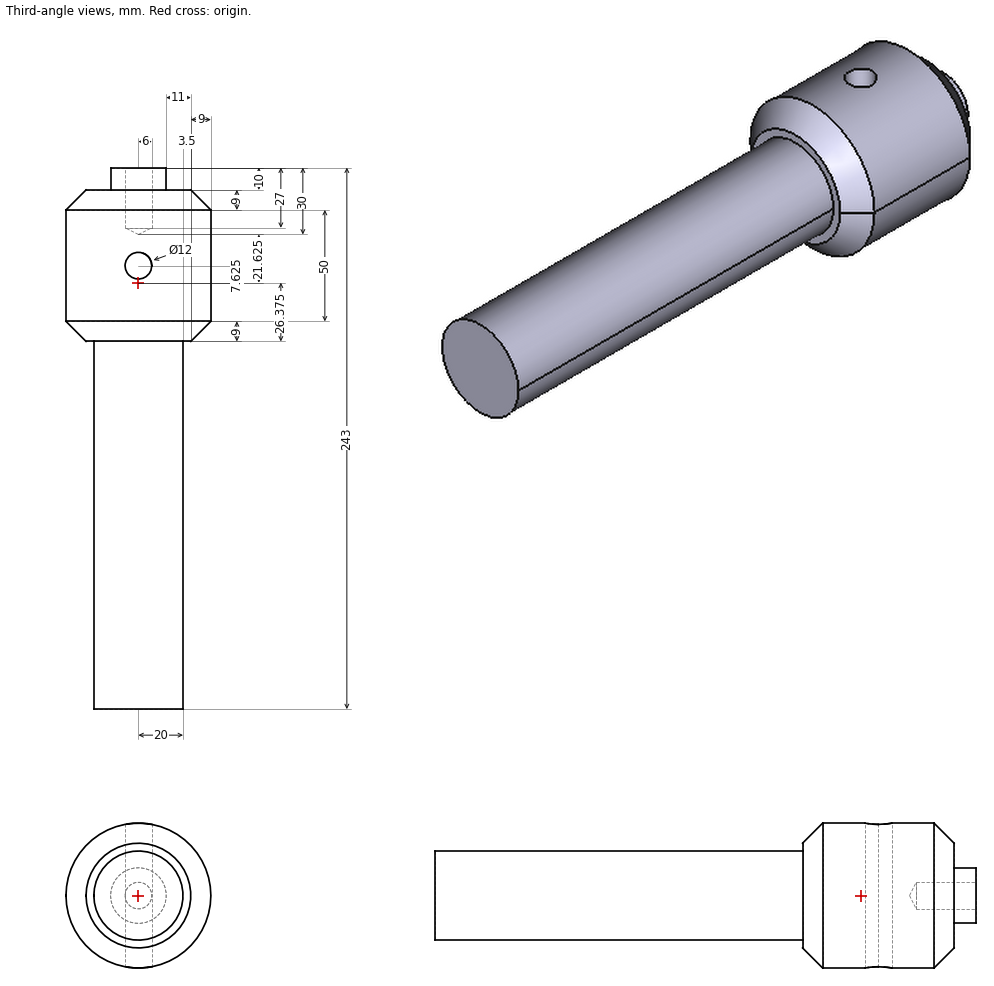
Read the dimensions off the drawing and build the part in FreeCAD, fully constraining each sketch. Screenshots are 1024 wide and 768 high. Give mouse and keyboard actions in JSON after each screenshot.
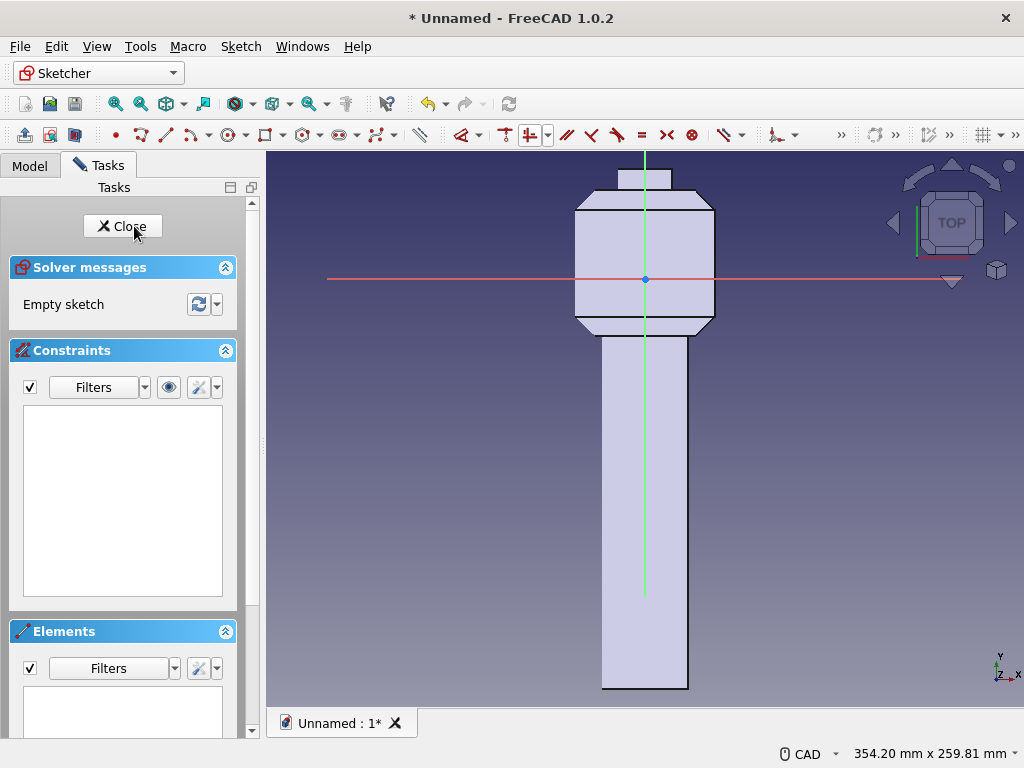
{"action": "scroll", "coordinate": [576, 429], "scroll_direction": "down", "scroll_amount": 5}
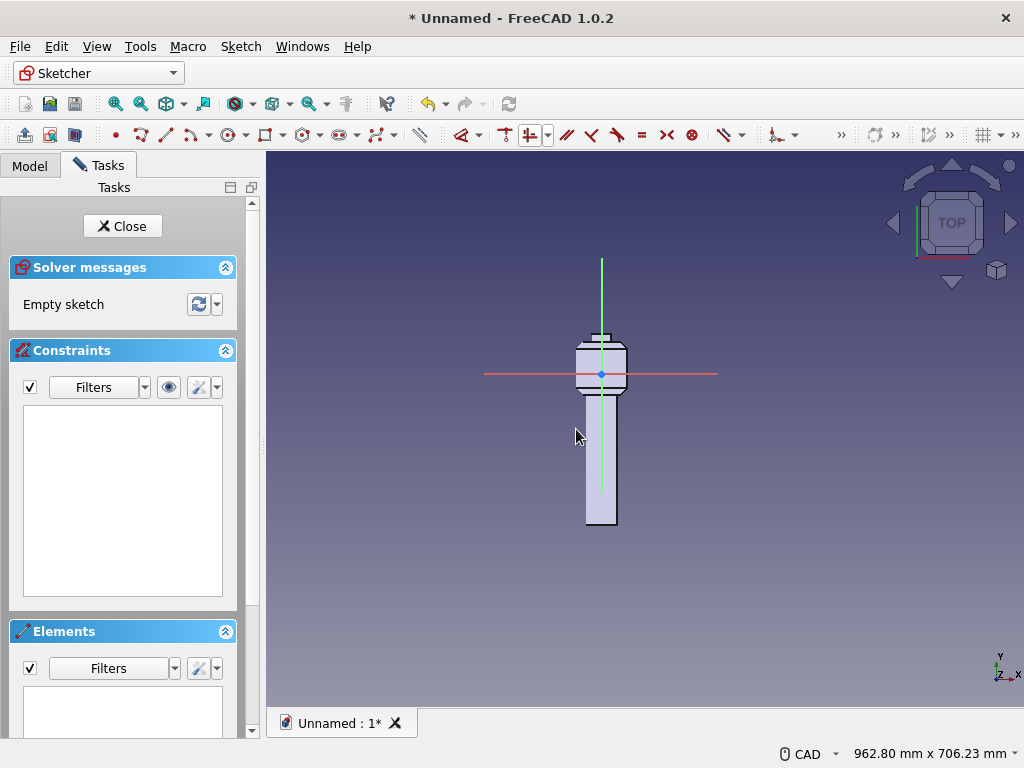
{"action": "scroll", "coordinate": [607, 345], "scroll_direction": "up", "scroll_amount": 11}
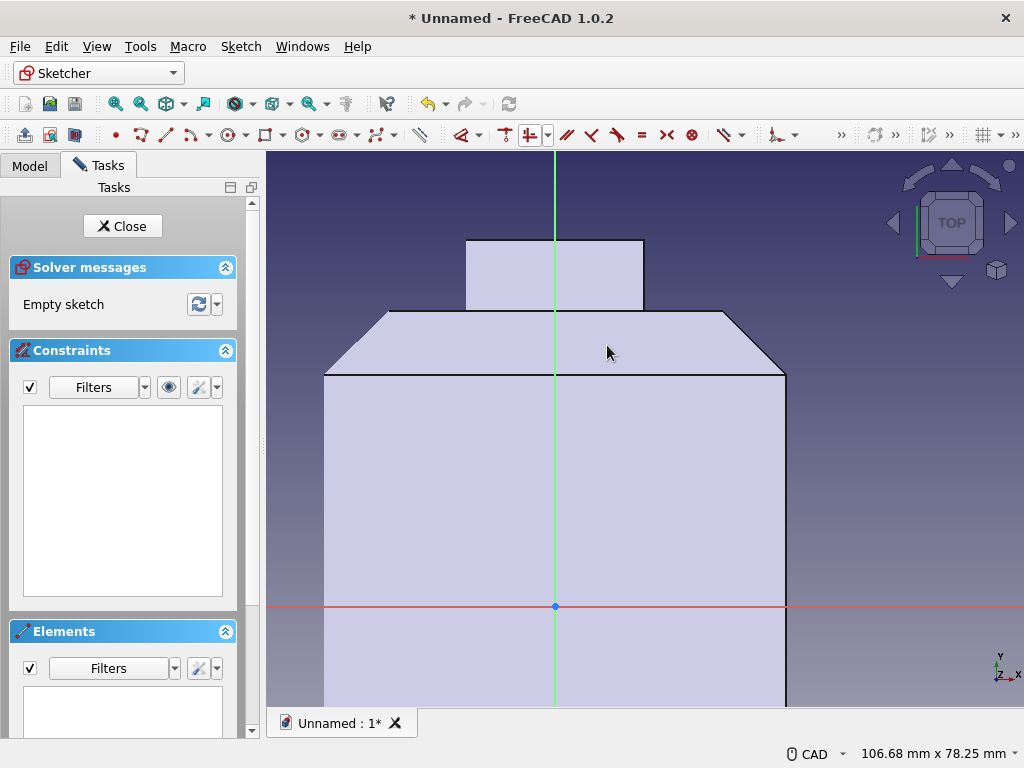
{"action": "left_click", "coordinate": [141, 136]}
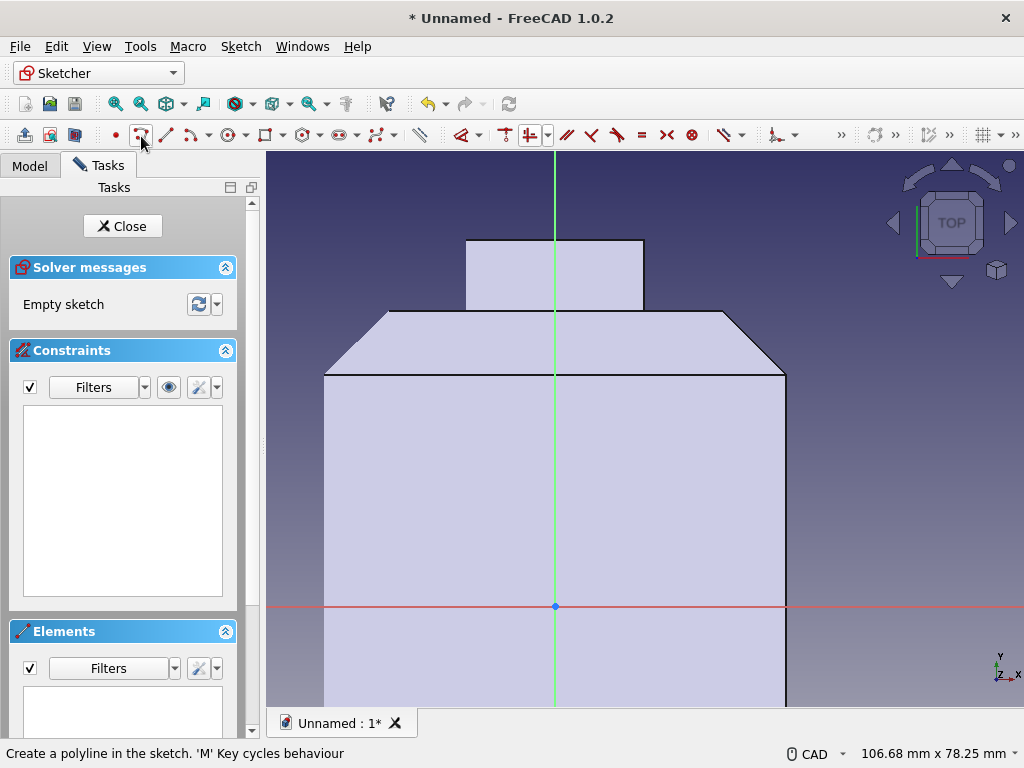
{"action": "left_click", "coordinate": [555, 453]}
{"action": "left_click", "coordinate": [598, 432]}
{"action": "left_click", "coordinate": [598, 240]}
{"action": "left_click", "coordinate": [564, 240]}
{"action": "left_click", "coordinate": [555, 454]}
{"action": "key", "text": "Escape"}
{"action": "key", "text": "Escape"}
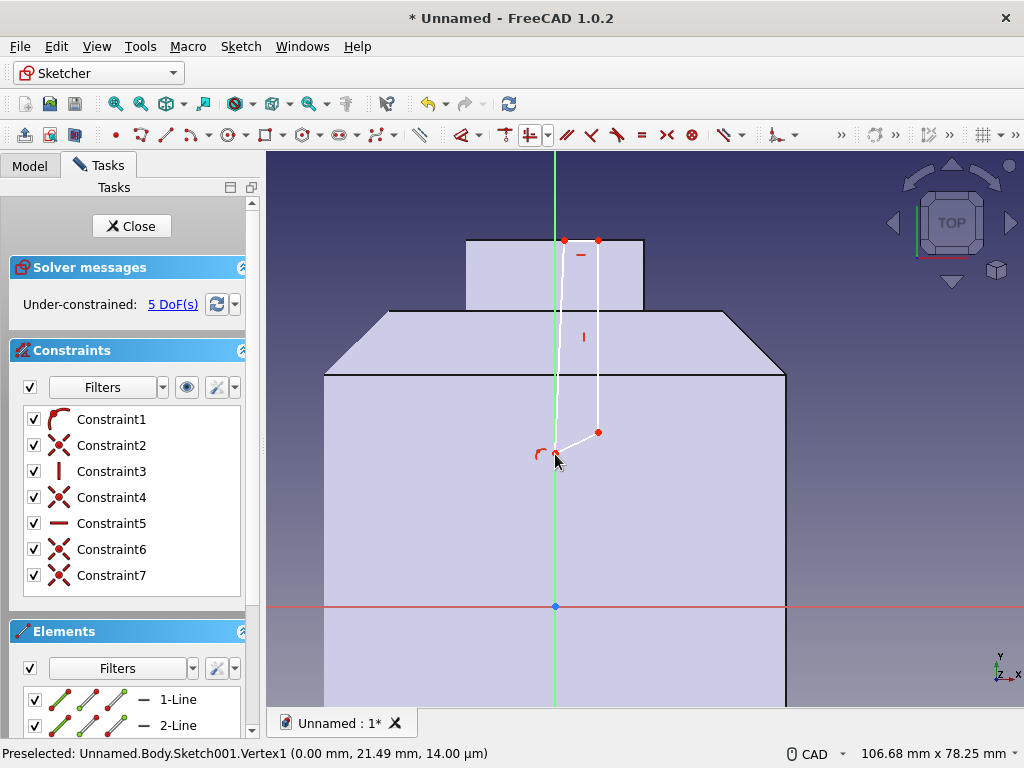
{"action": "left_click", "coordinate": [558, 390]}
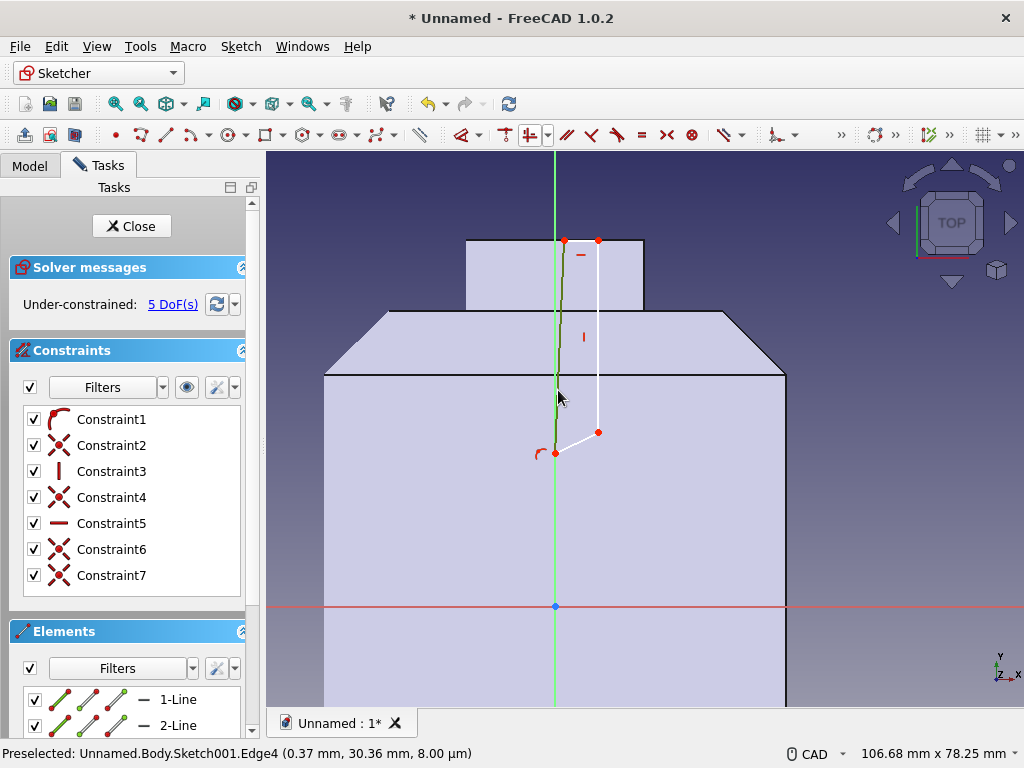
{"action": "left_click", "coordinate": [548, 136]}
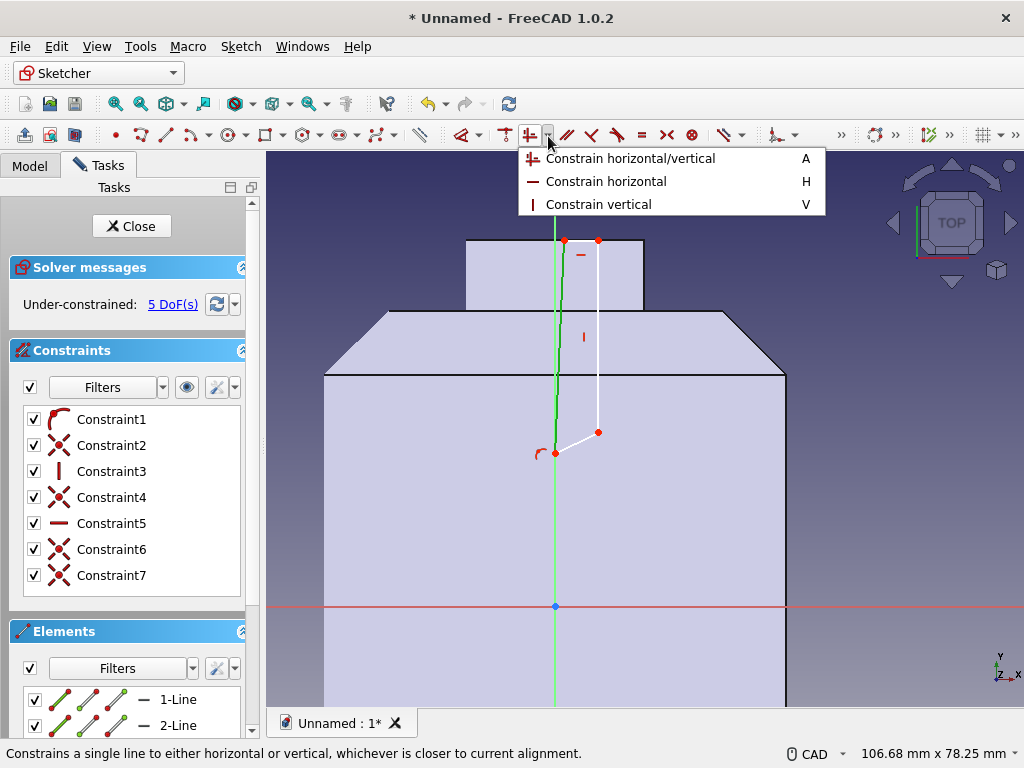
{"action": "left_click", "coordinate": [672, 204]}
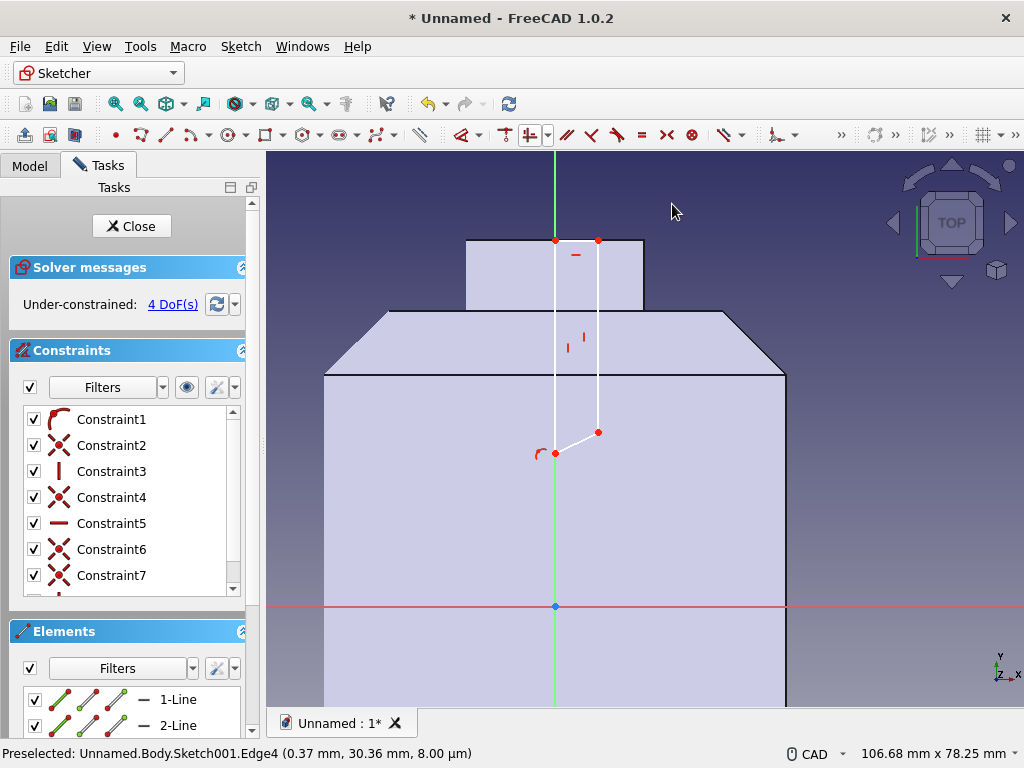
{"action": "left_click", "coordinate": [460, 136]}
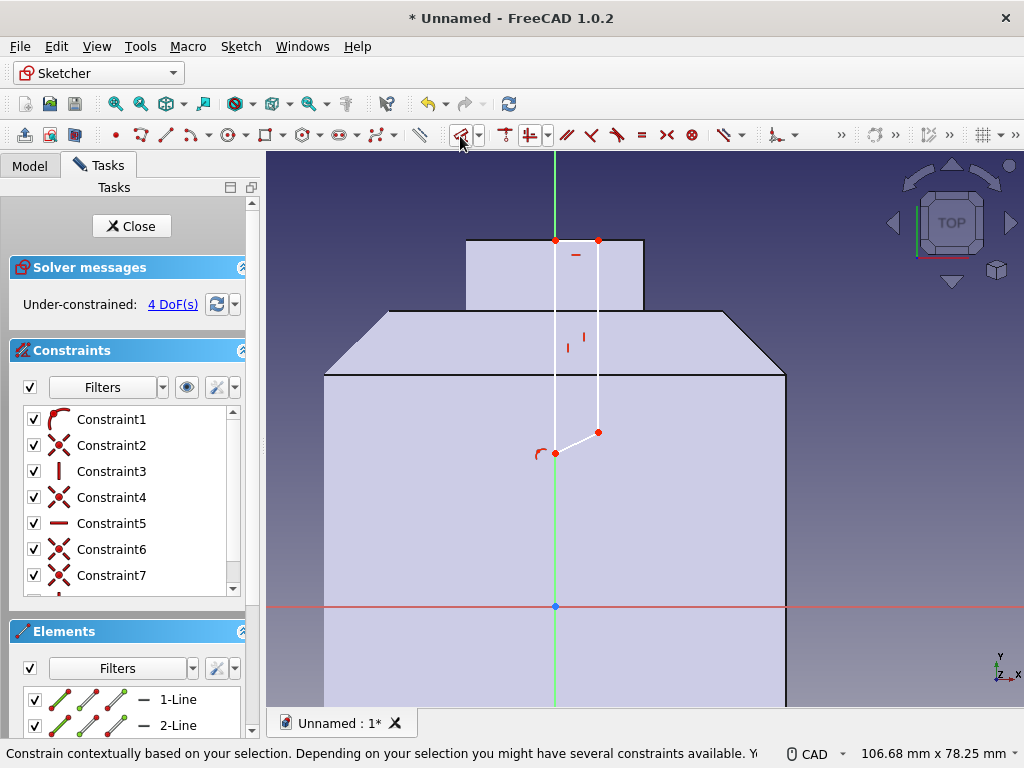
{"action": "left_click", "coordinate": [585, 241]}
{"action": "left_click", "coordinate": [577, 207]}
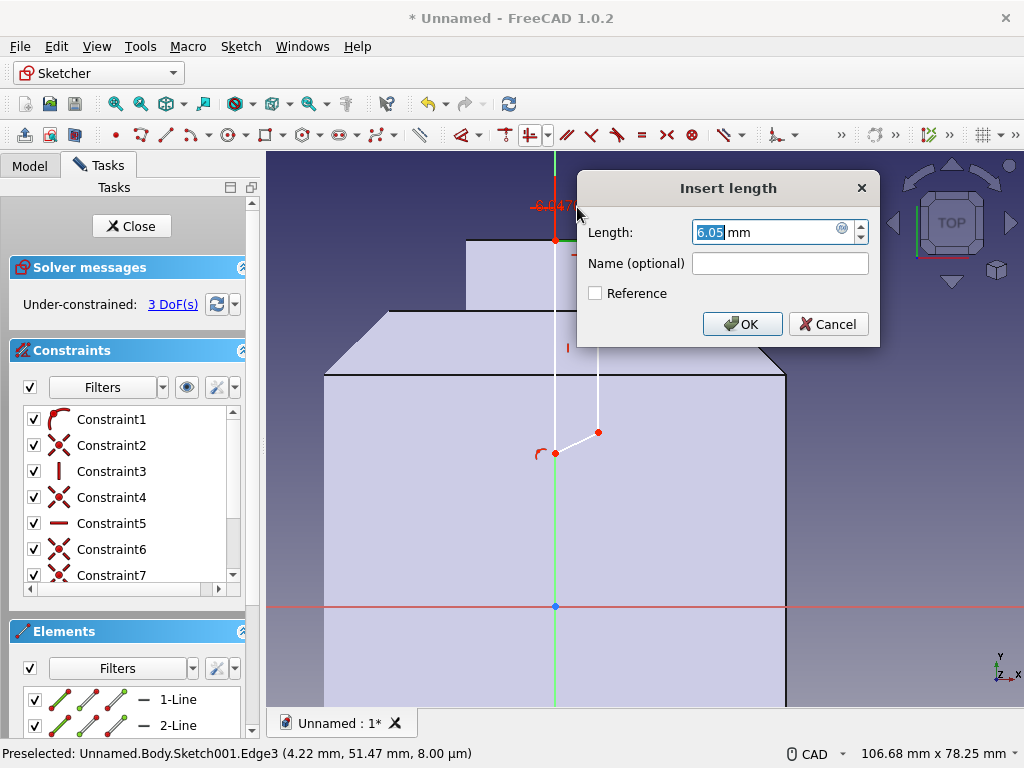
{"action": "type", "text": "6"}
{"action": "key", "text": "Return"}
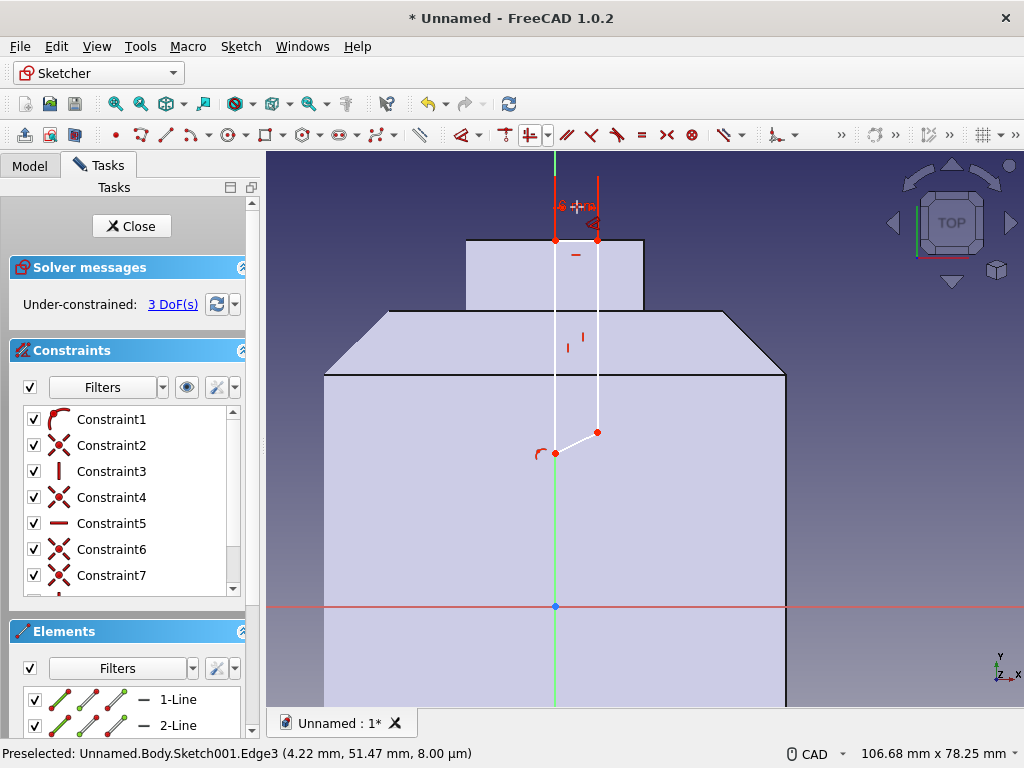
{"action": "left_click", "coordinate": [598, 375]}
{"action": "left_click", "coordinate": [632, 337]}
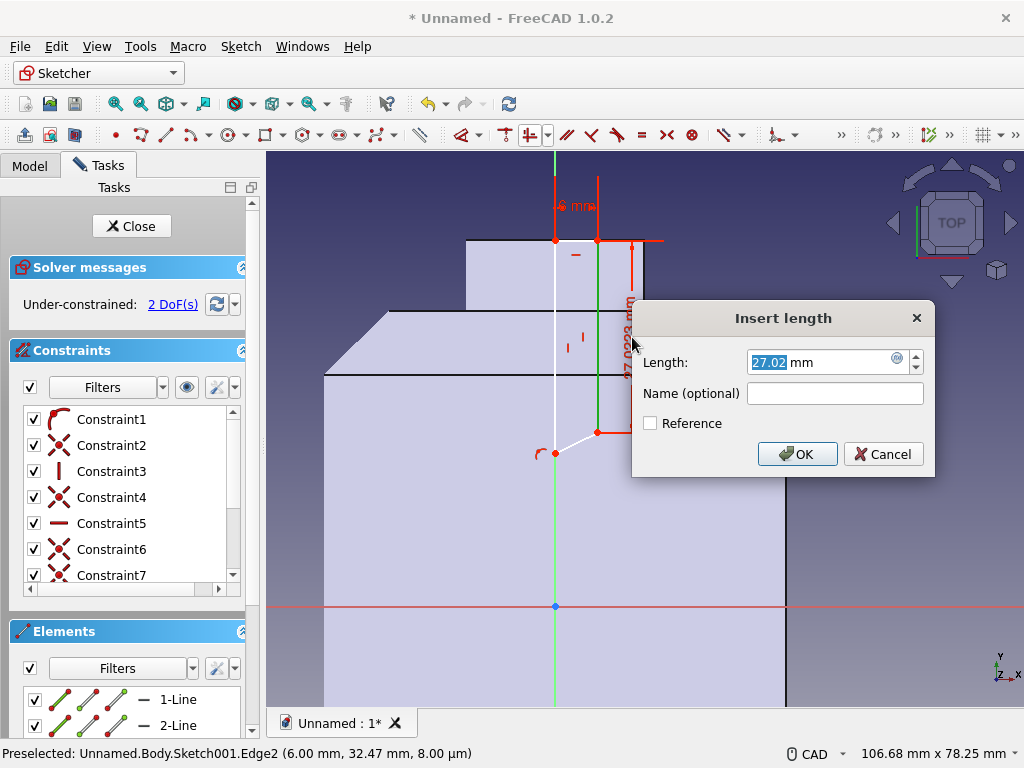
{"action": "type", "text": "27"}
{"action": "key", "text": "Return"}